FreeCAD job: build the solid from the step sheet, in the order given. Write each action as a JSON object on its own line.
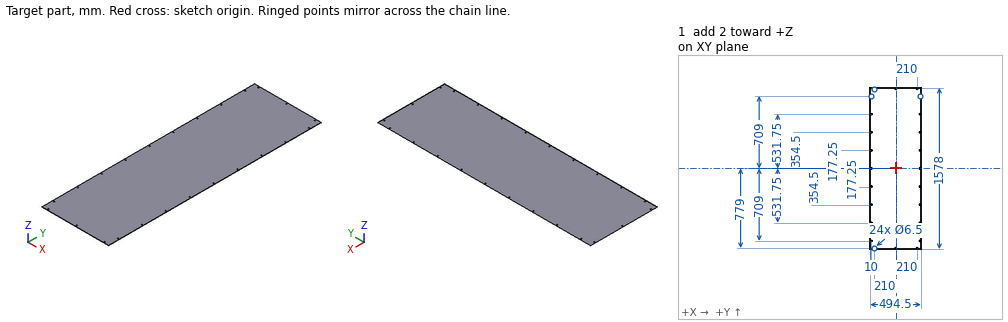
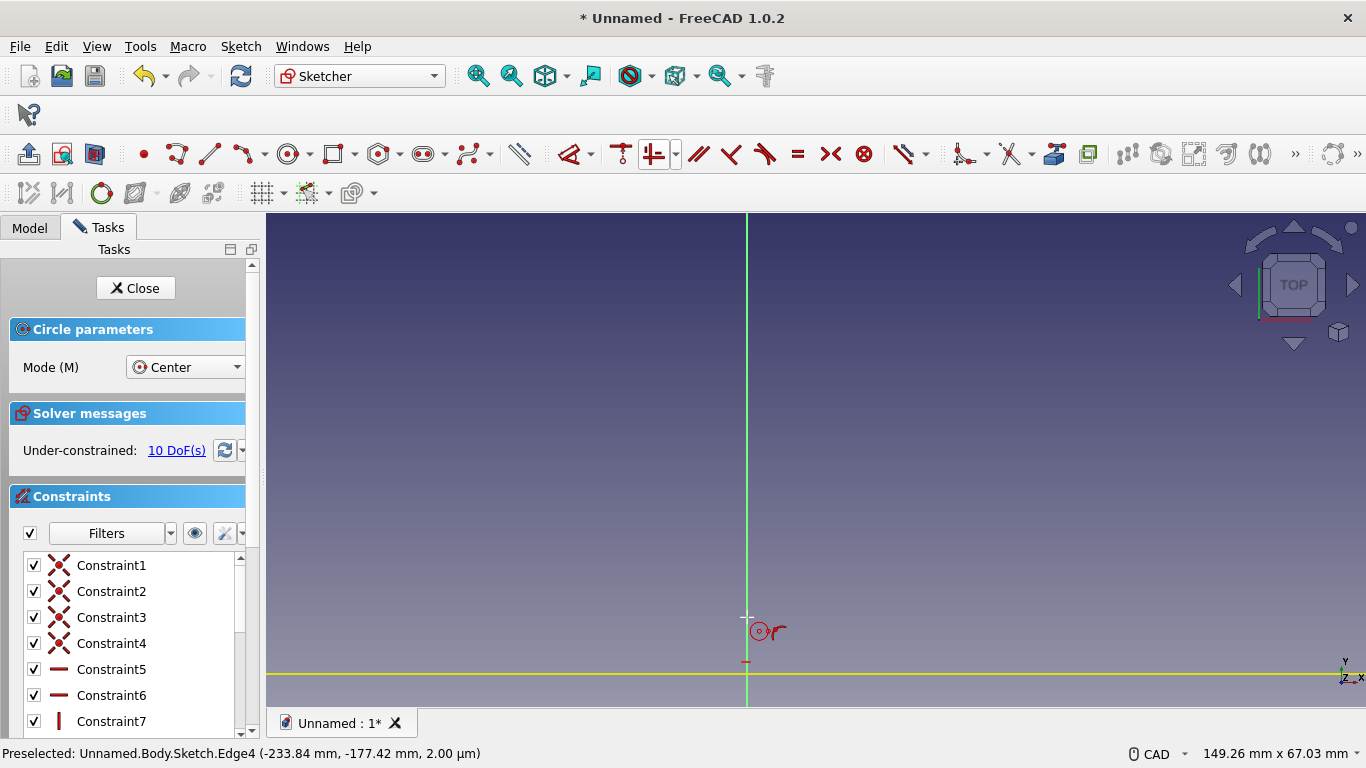
{"action": "scroll", "coordinate": [748, 617], "scroll_direction": "down", "scroll_amount": 18}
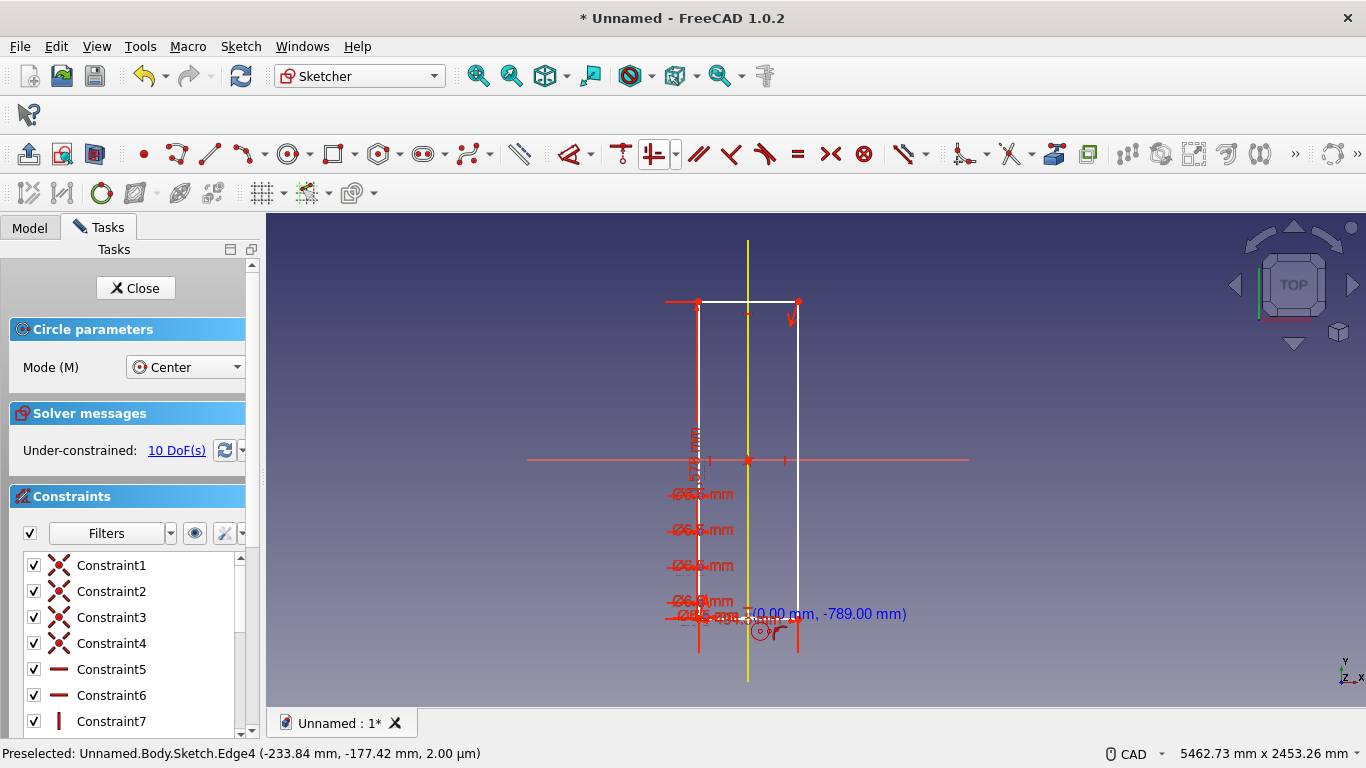
{"action": "scroll", "coordinate": [748, 617], "scroll_direction": "up", "scroll_amount": 11}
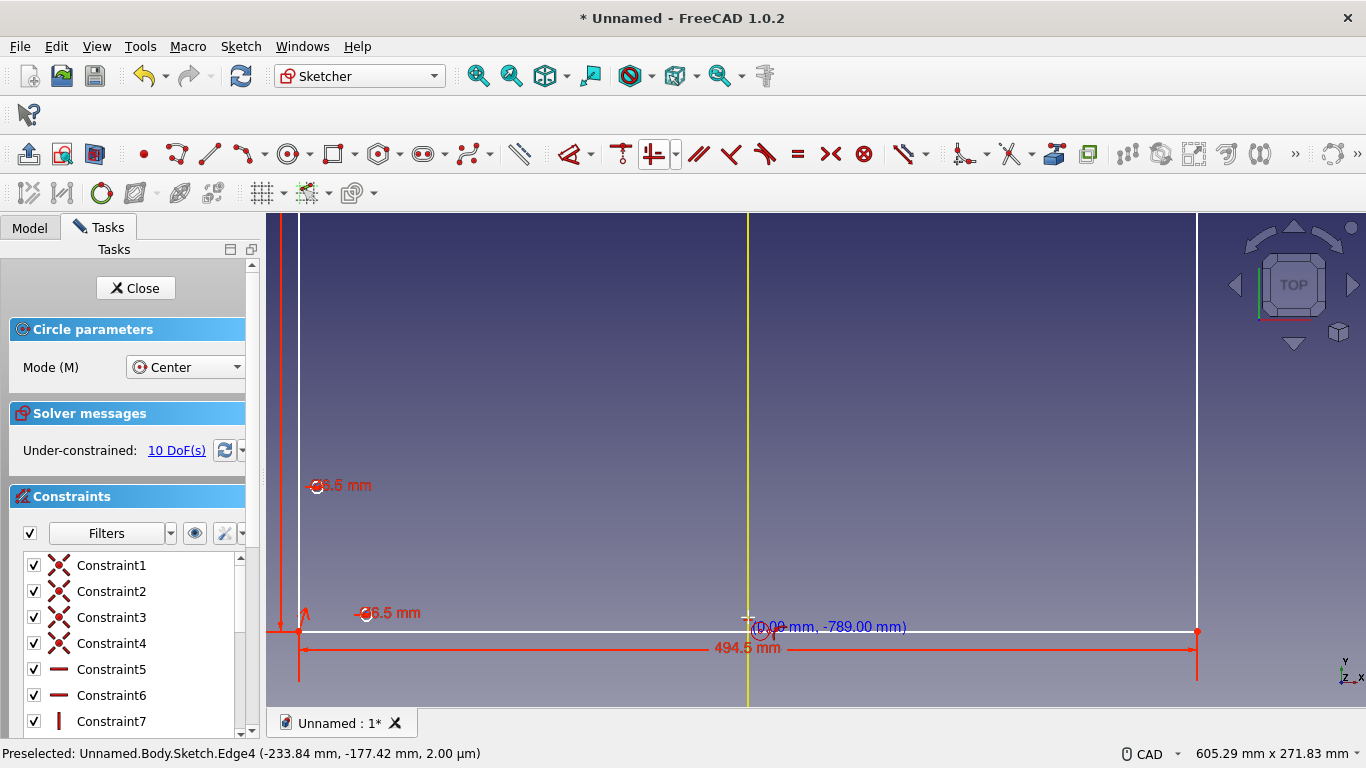
{"action": "left_click", "coordinate": [748, 614]}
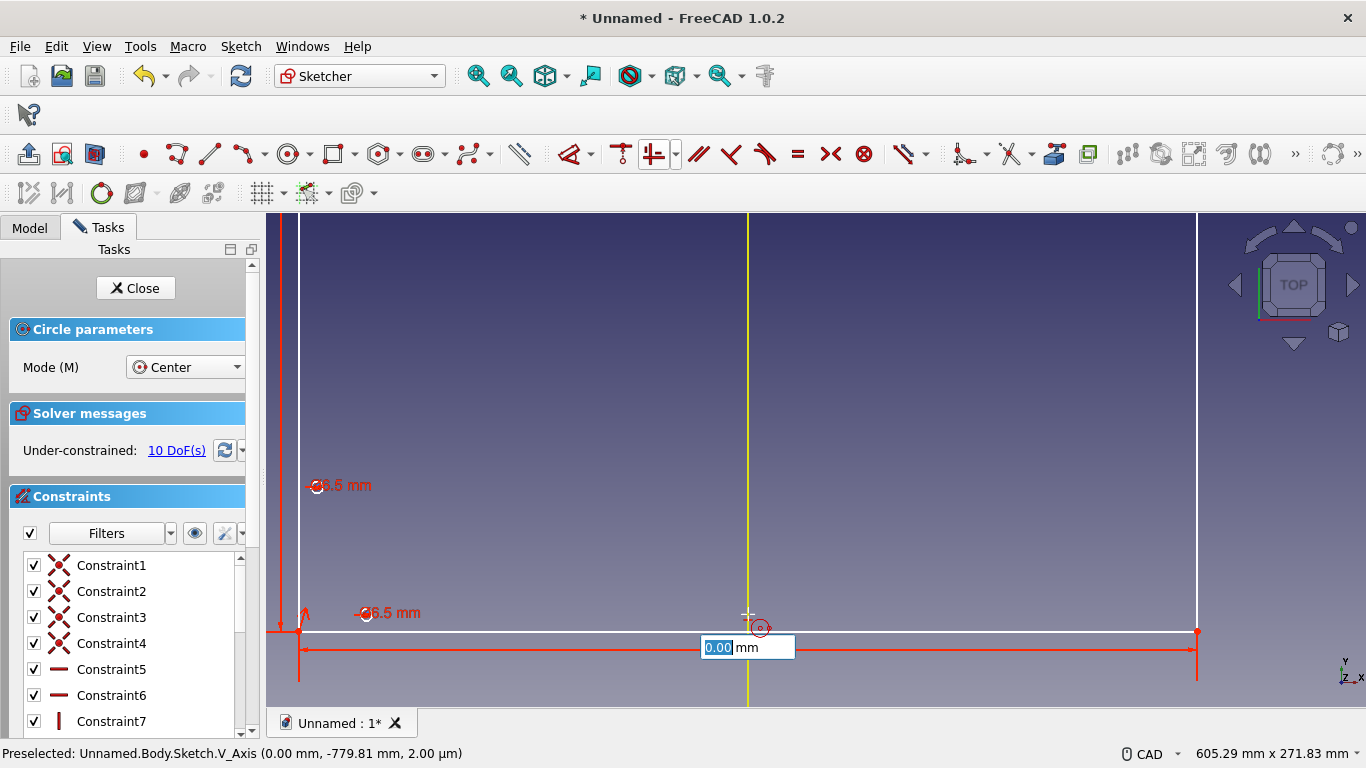
{"action": "scroll", "coordinate": [754, 612], "scroll_direction": "up", "scroll_amount": 6}
{"action": "mouse_move", "coordinate": [752, 608]}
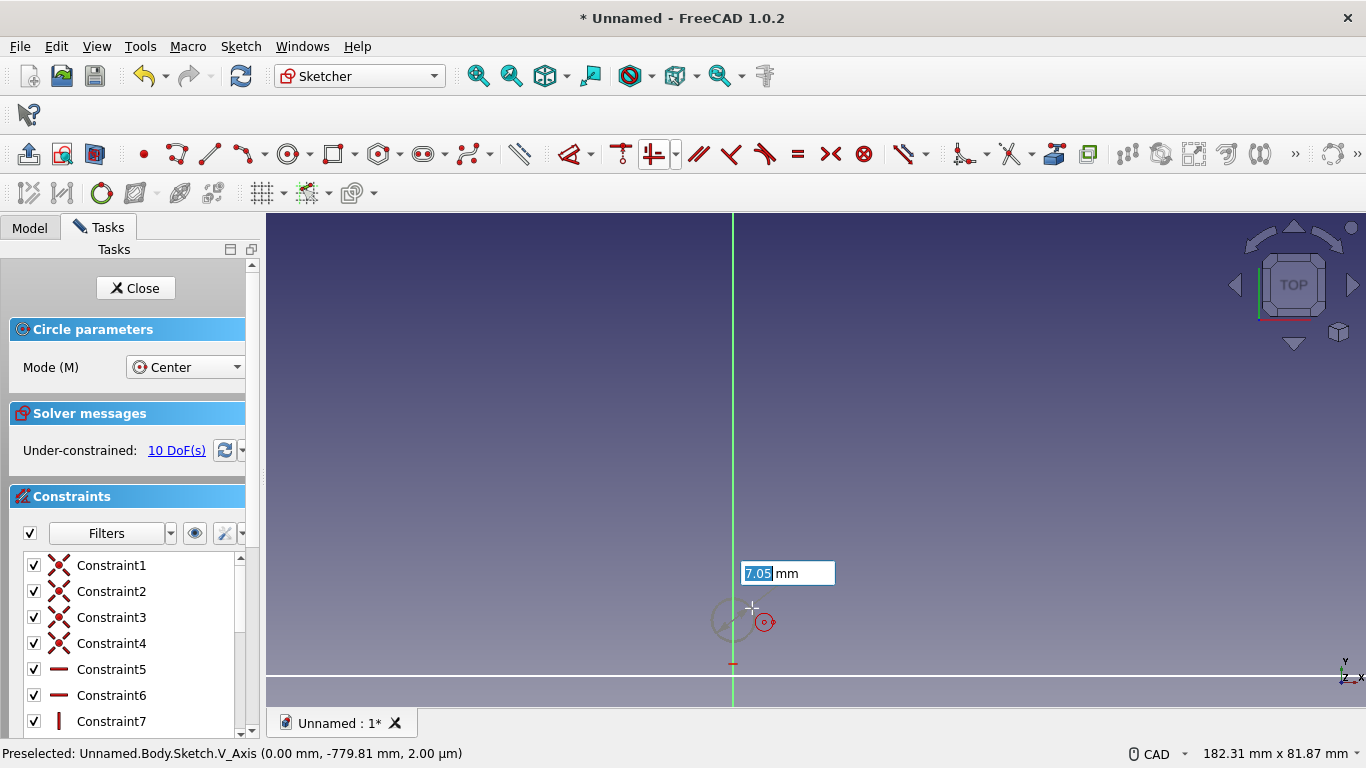
{"action": "type", "text": "6.5"}
{"action": "key", "text": "Return"}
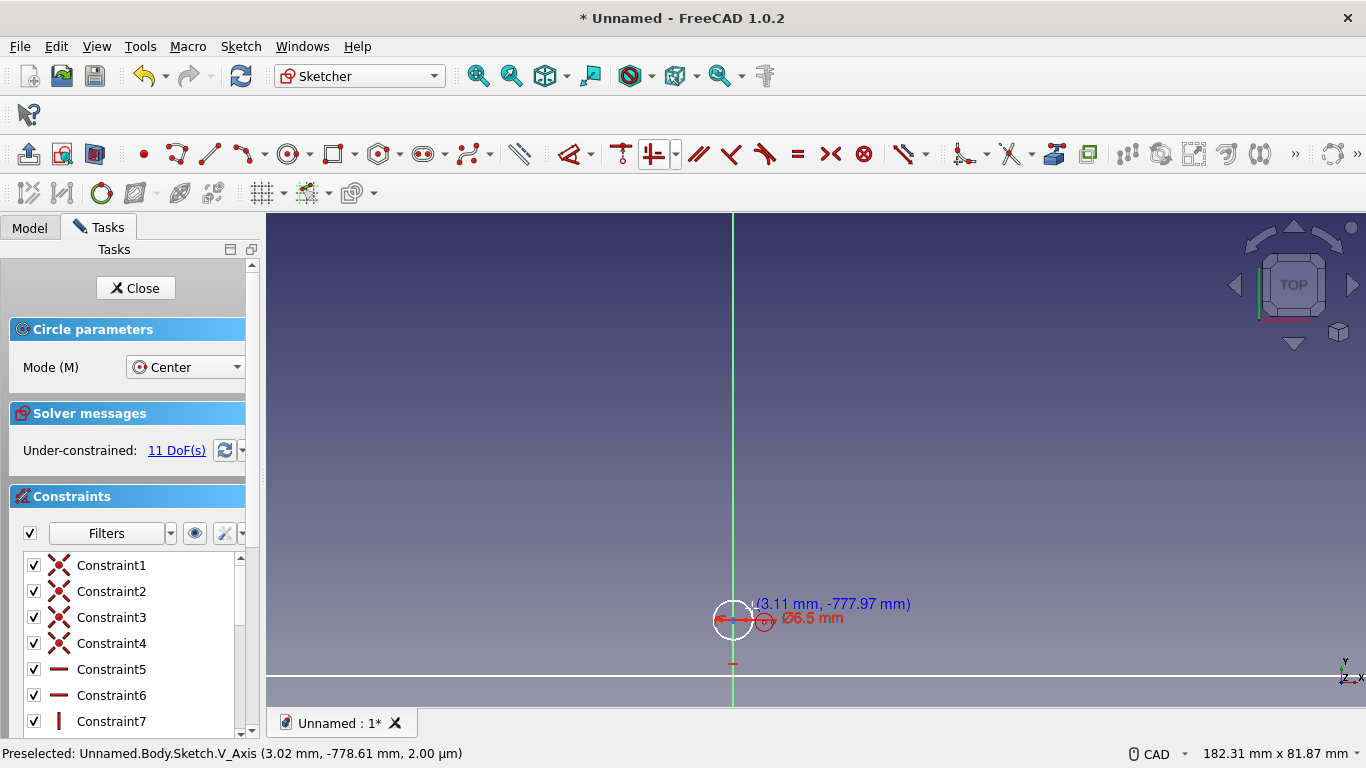
{"action": "scroll", "coordinate": [748, 617], "scroll_direction": "down", "scroll_amount": 17}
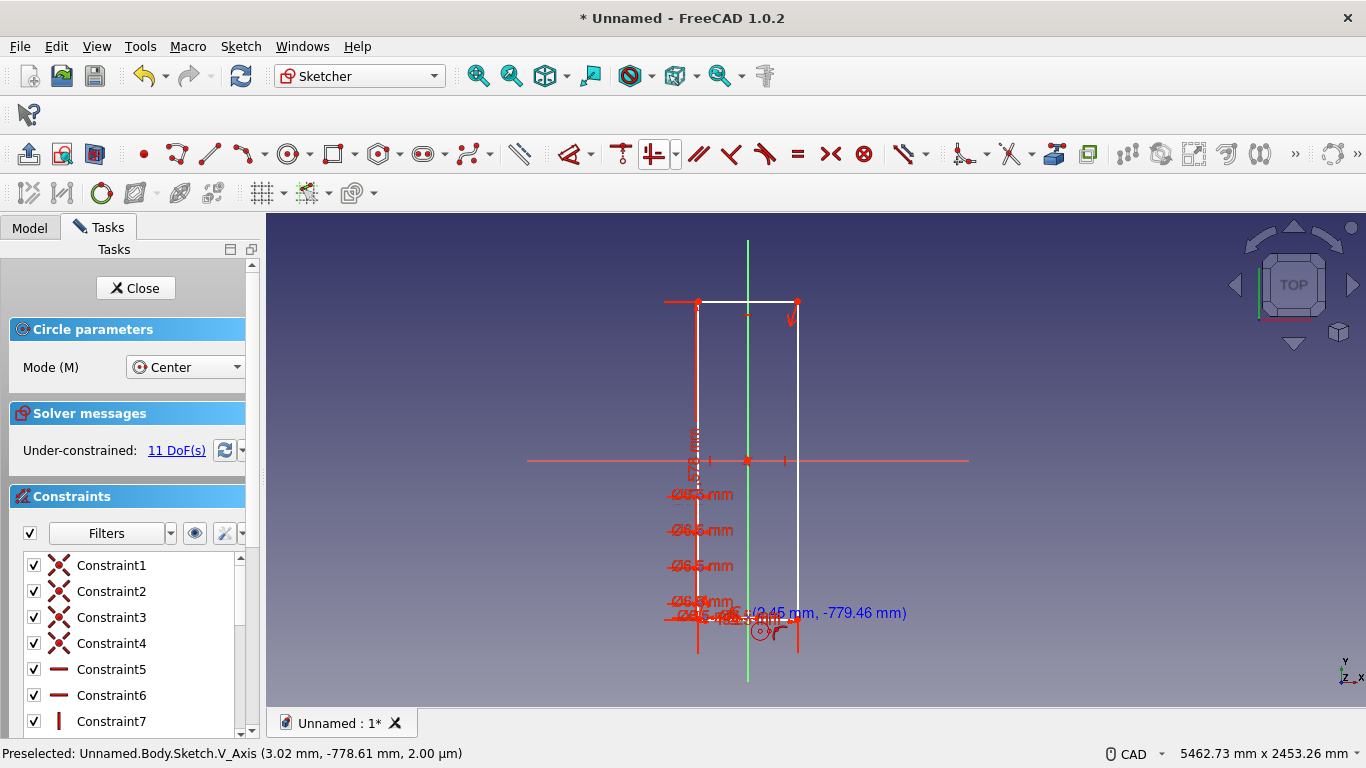
{"action": "scroll", "coordinate": [790, 618], "scroll_direction": "up", "scroll_amount": 18}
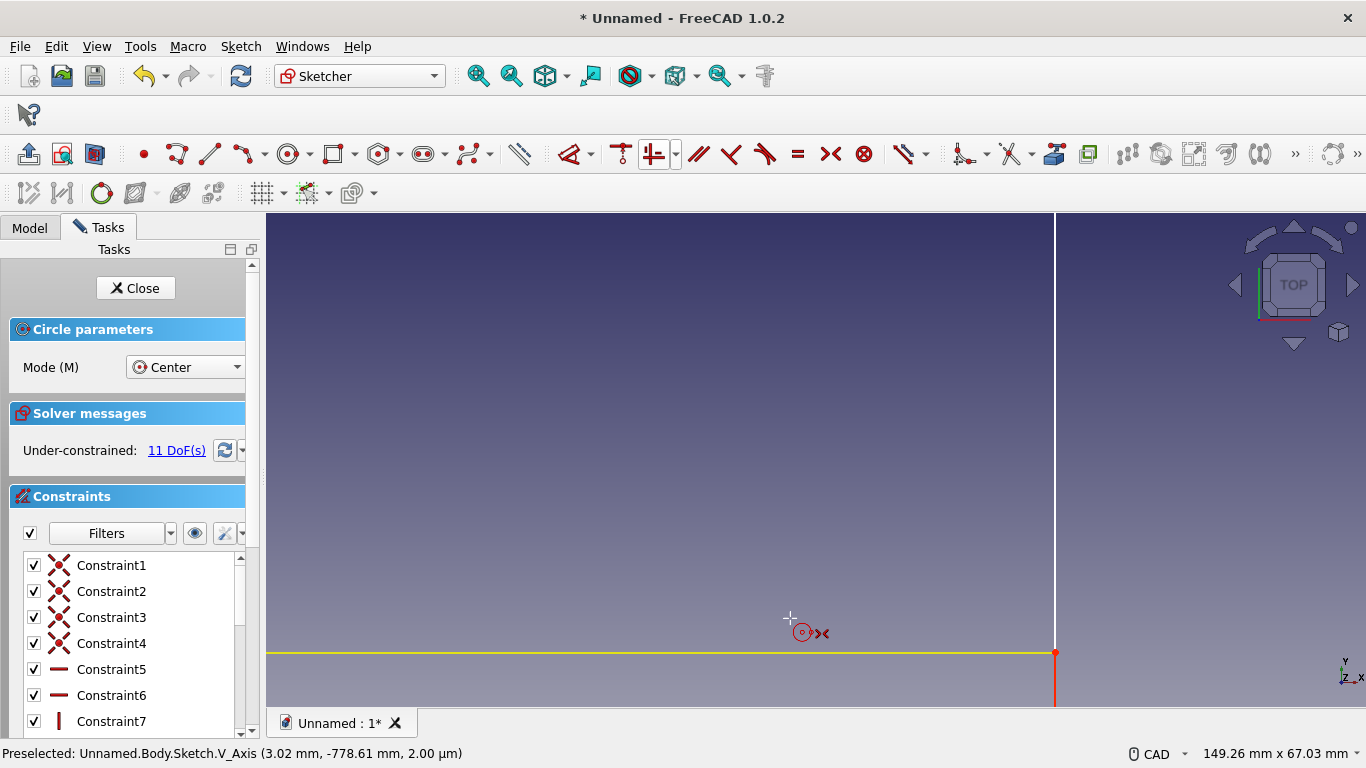
{"action": "scroll", "coordinate": [790, 618], "scroll_direction": "down", "scroll_amount": 18}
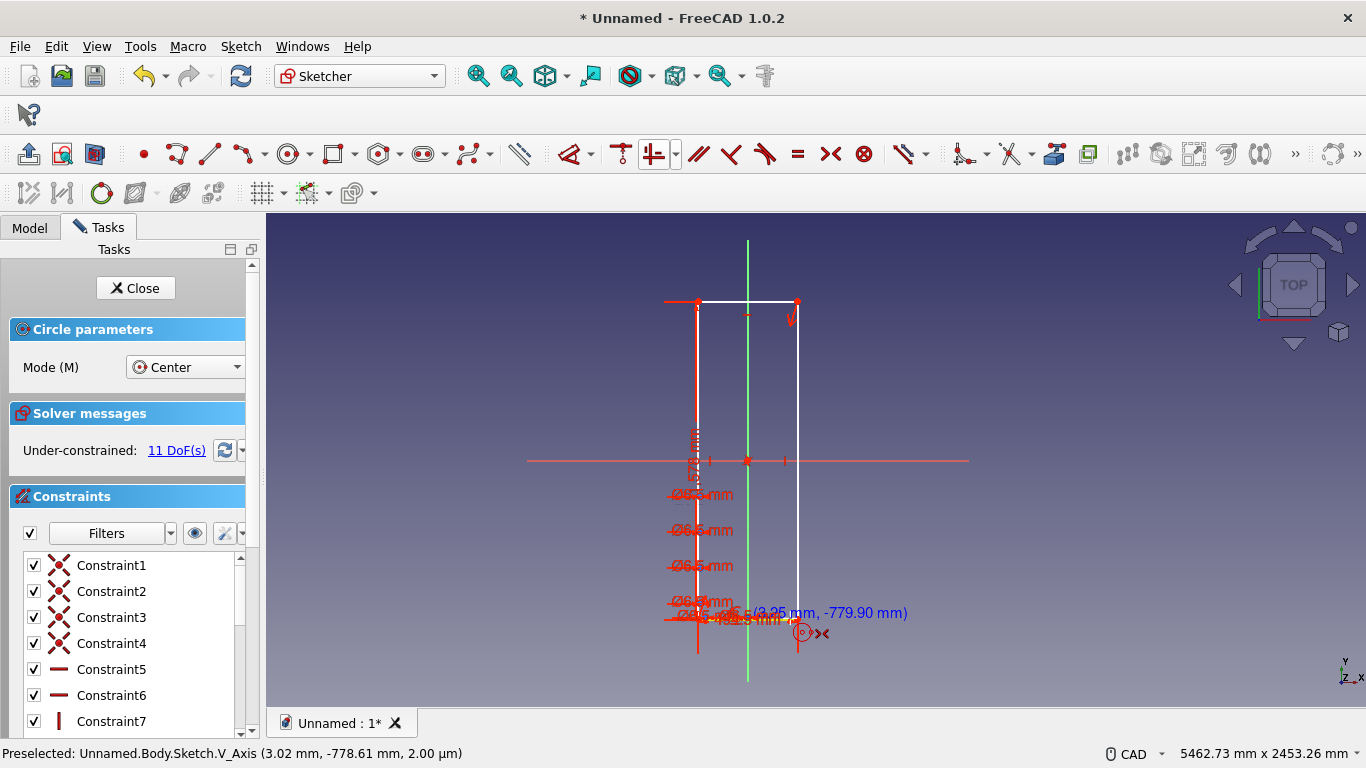
{"action": "scroll", "coordinate": [790, 618], "scroll_direction": "up", "scroll_amount": 11}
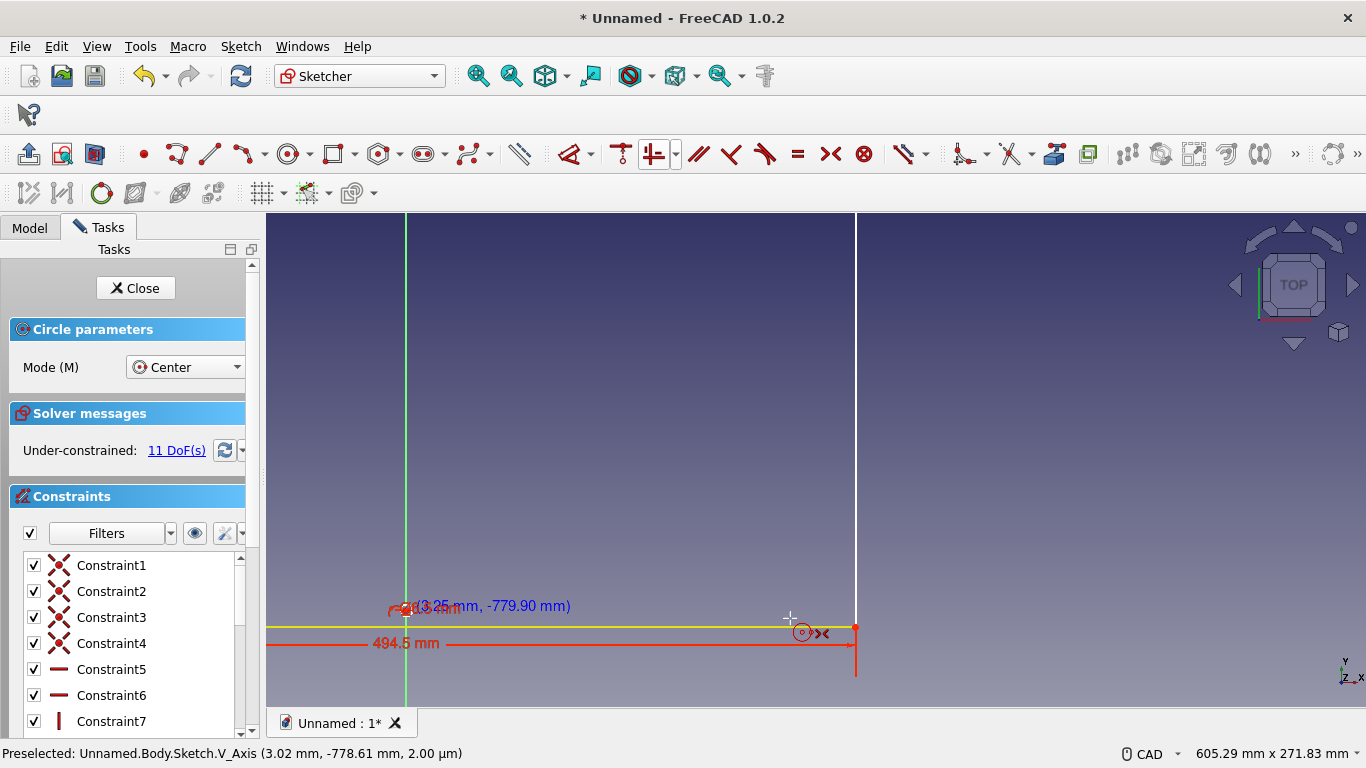
{"action": "left_click", "coordinate": [788, 609]}
{"action": "mouse_move", "coordinate": [792, 605]}